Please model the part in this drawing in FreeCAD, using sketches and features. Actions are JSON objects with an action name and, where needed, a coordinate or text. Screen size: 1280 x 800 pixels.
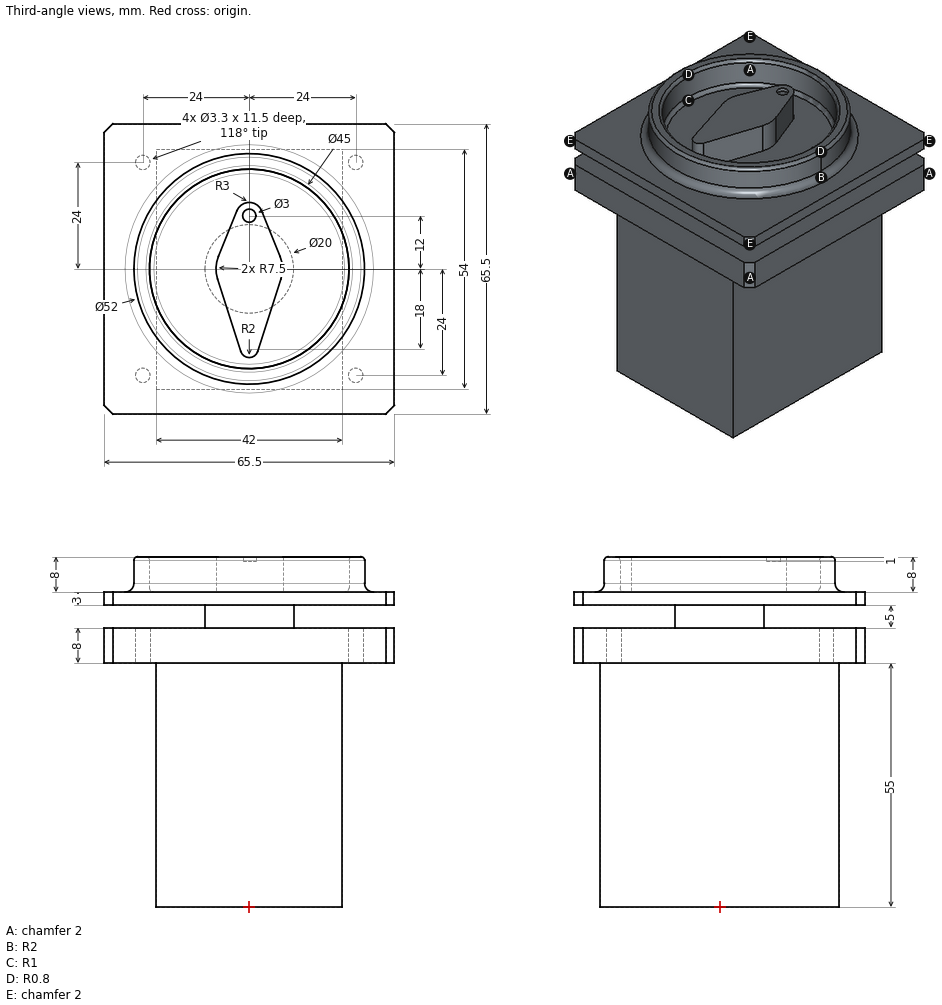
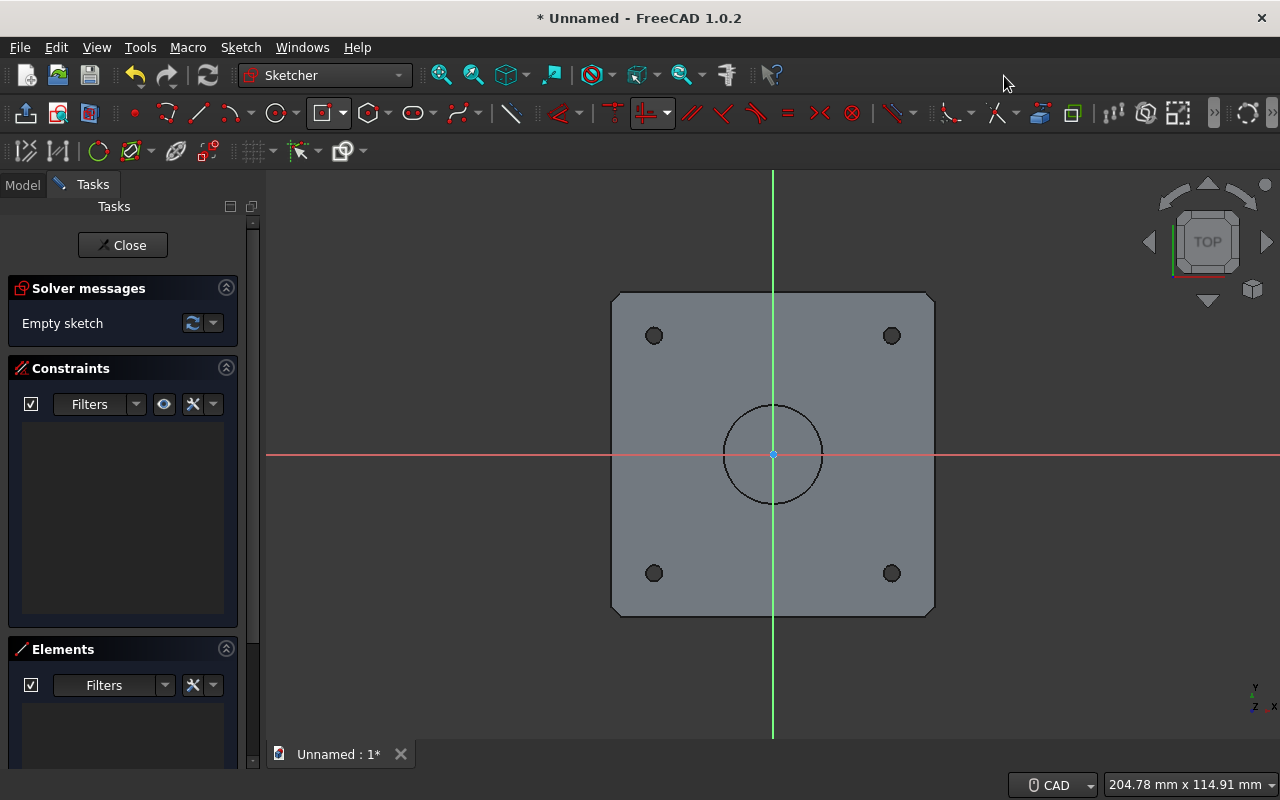
{"action": "left_click", "coordinate": [322, 114]}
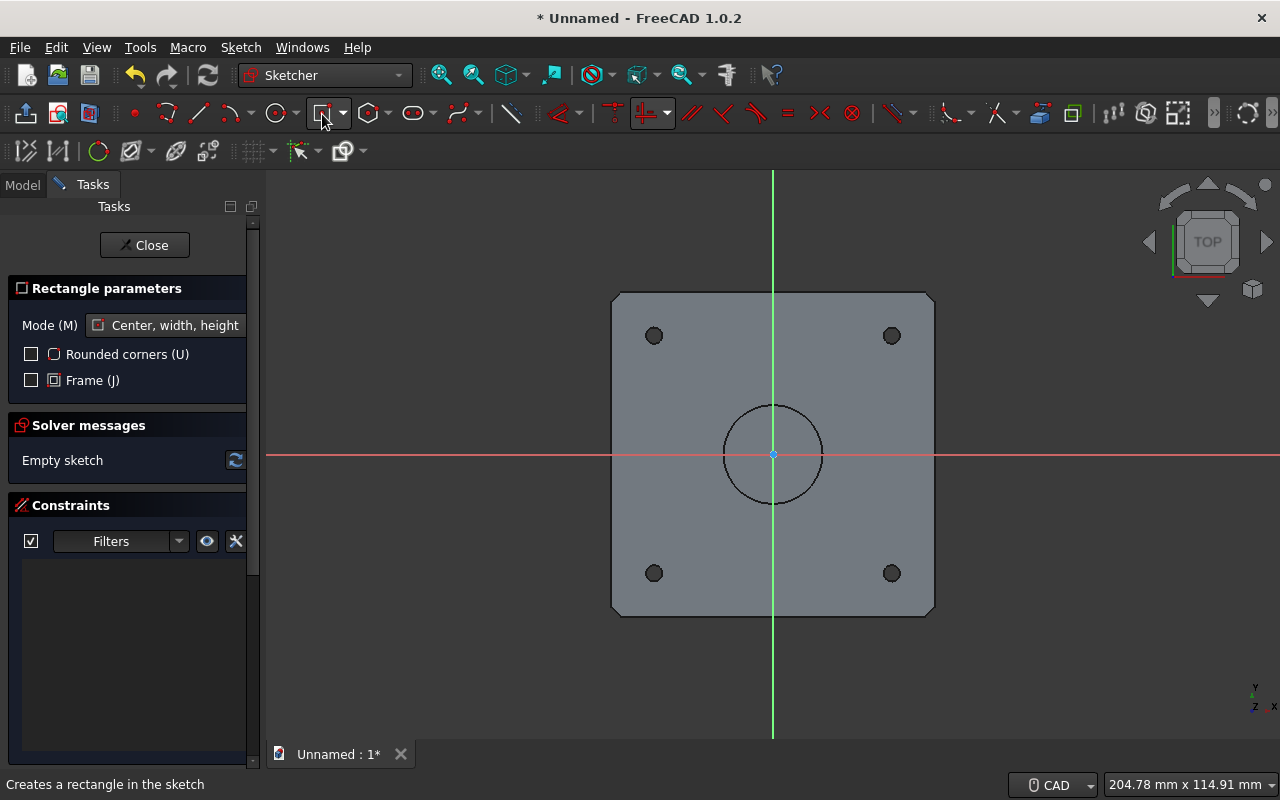
{"action": "left_click", "coordinate": [773, 455]}
{"action": "mouse_move", "coordinate": [935, 292]}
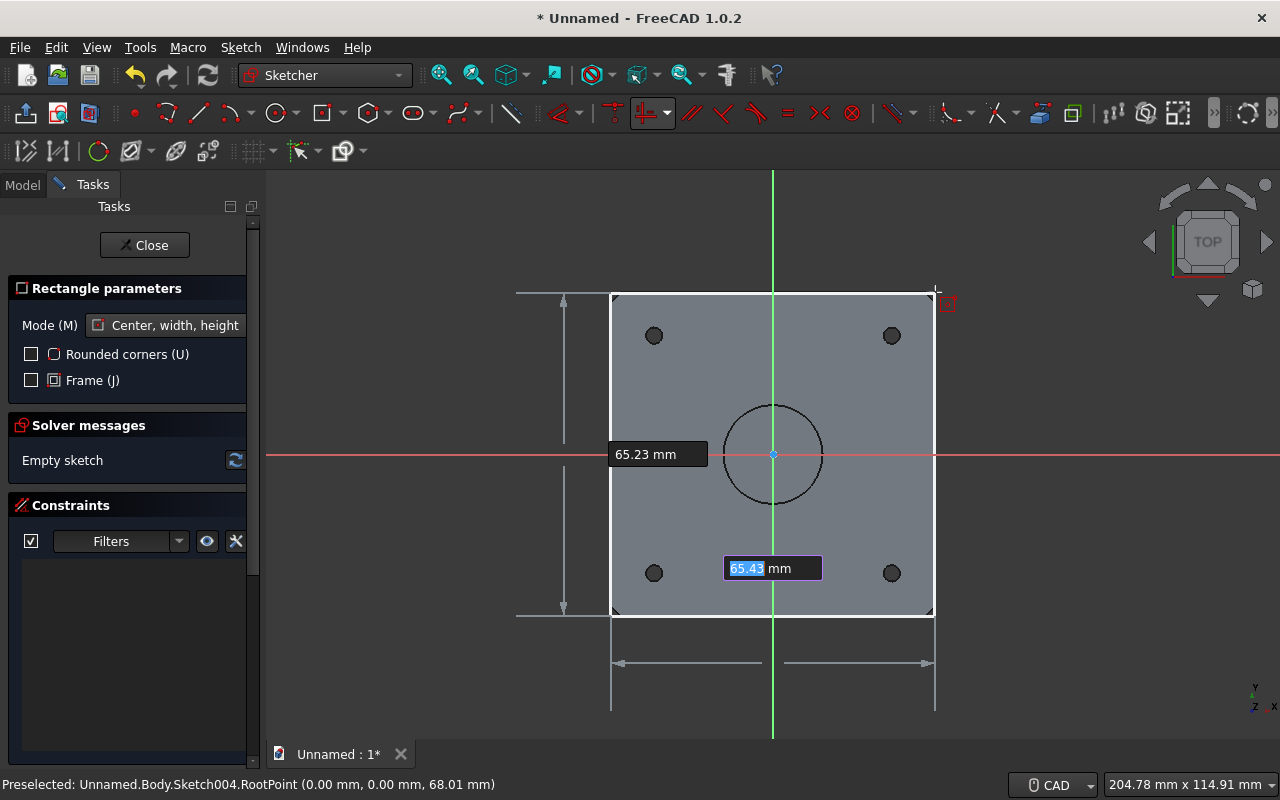
{"action": "type", "text": "65.5"}
{"action": "key", "text": "Tab"}
{"action": "type", "text": "65.5"}
{"action": "key", "text": "Return"}
{"action": "key", "text": "Escape"}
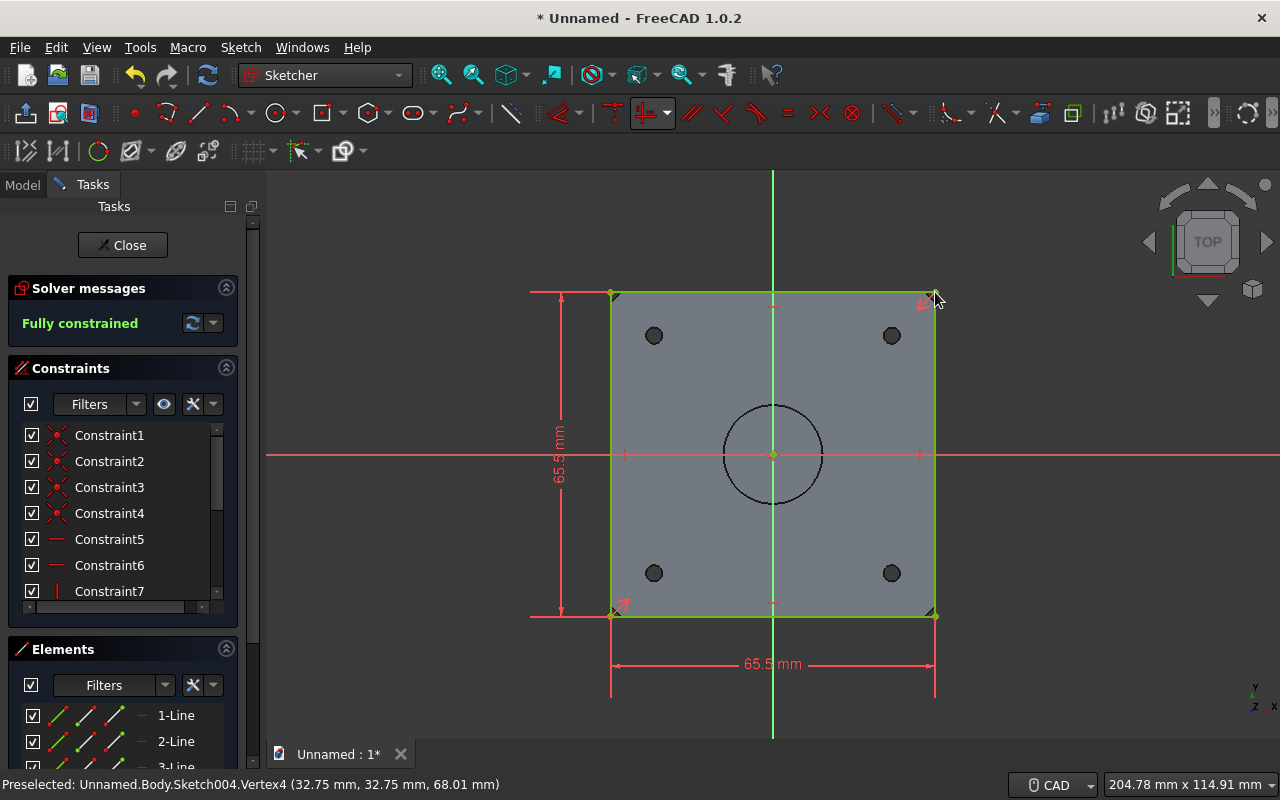
{"action": "left_click", "coordinate": [123, 245]}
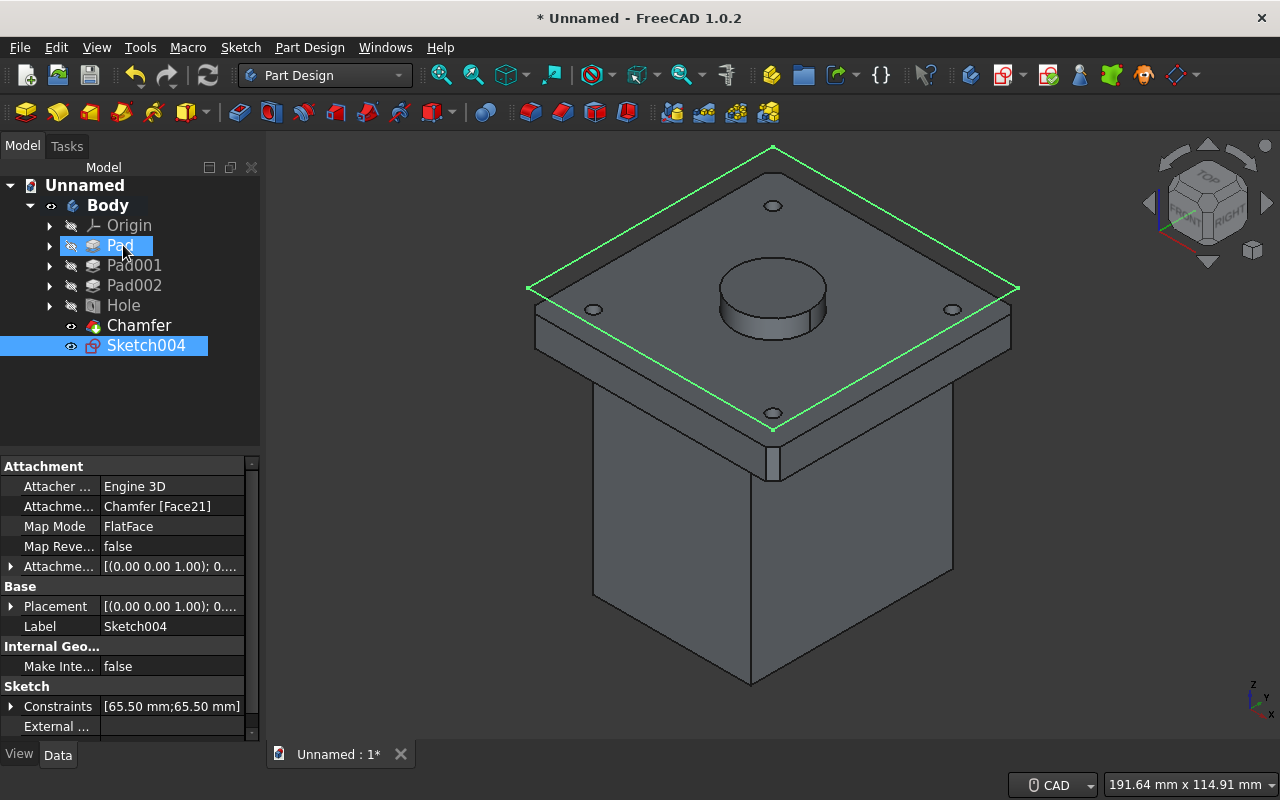
{"action": "left_click", "coordinate": [26, 112]}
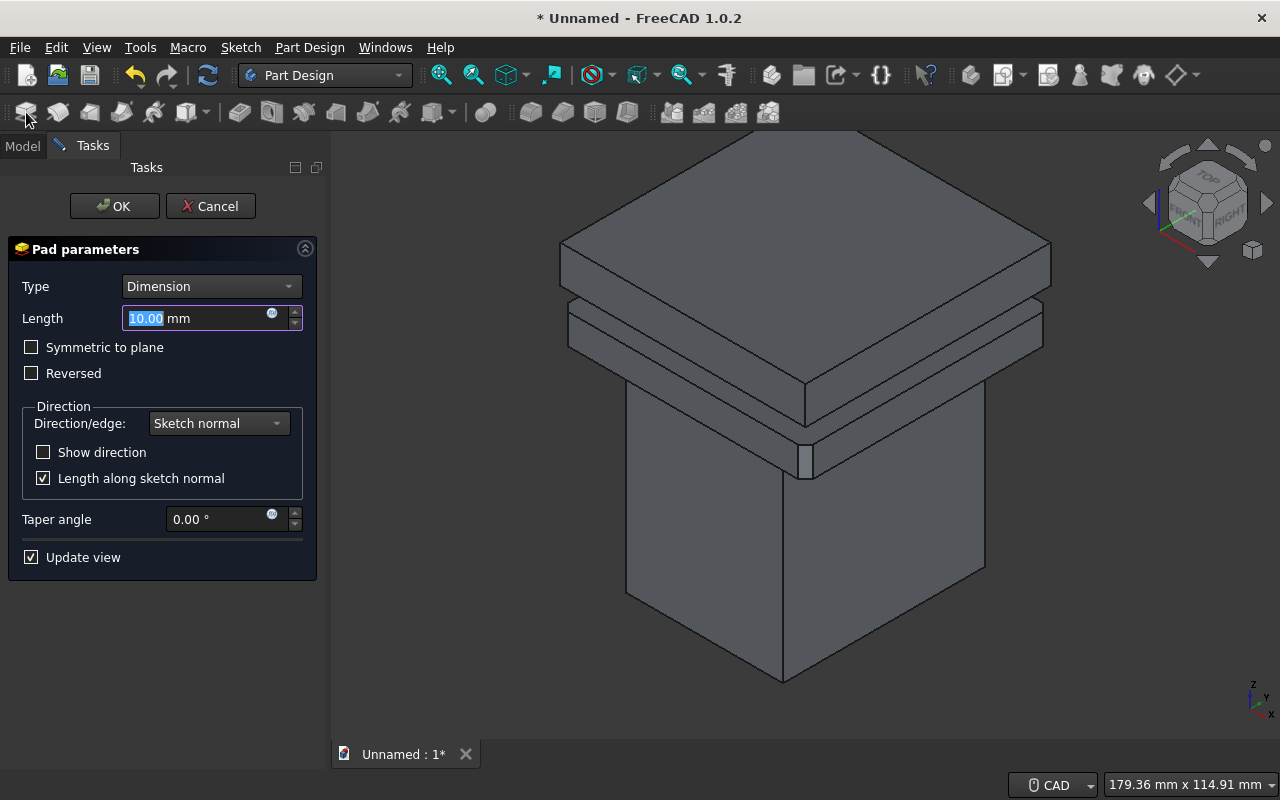
{"action": "type", "text": "3"}
{"action": "key", "text": "Tab"}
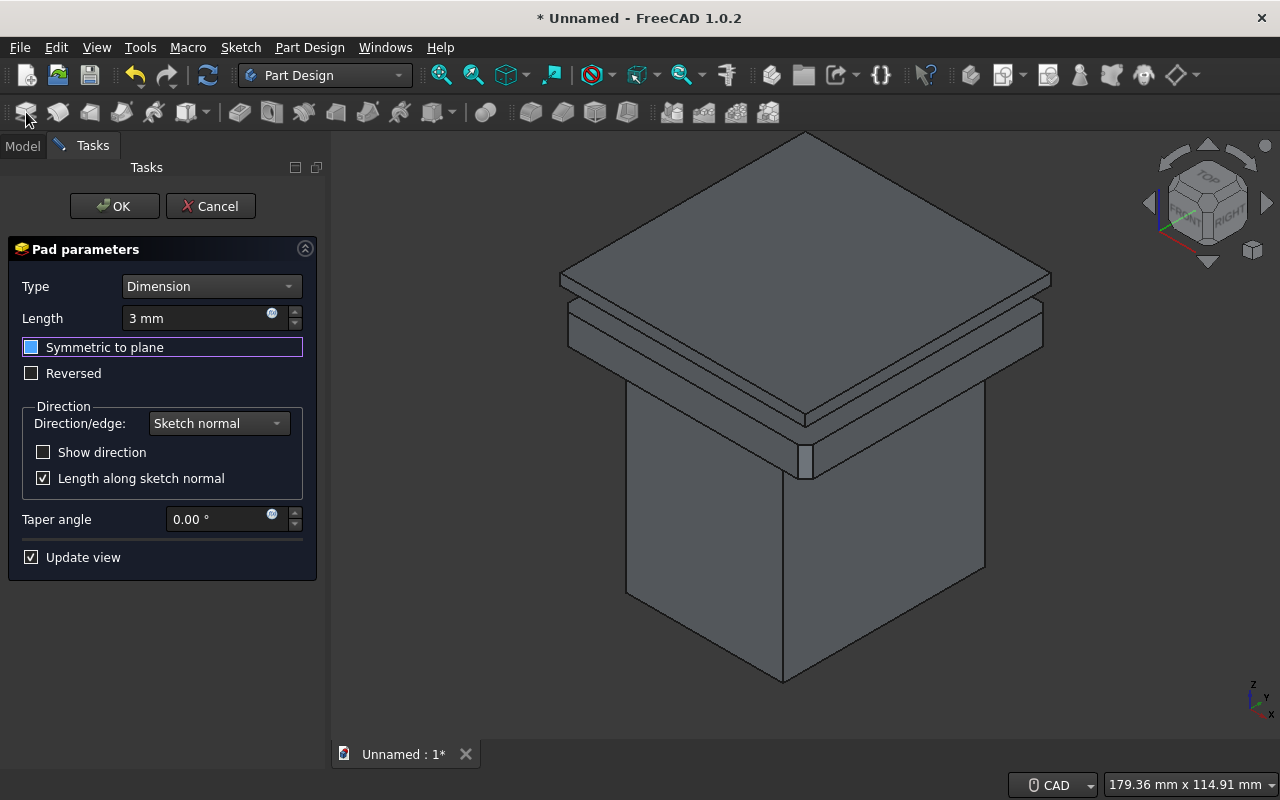
{"action": "left_click", "coordinate": [115, 206]}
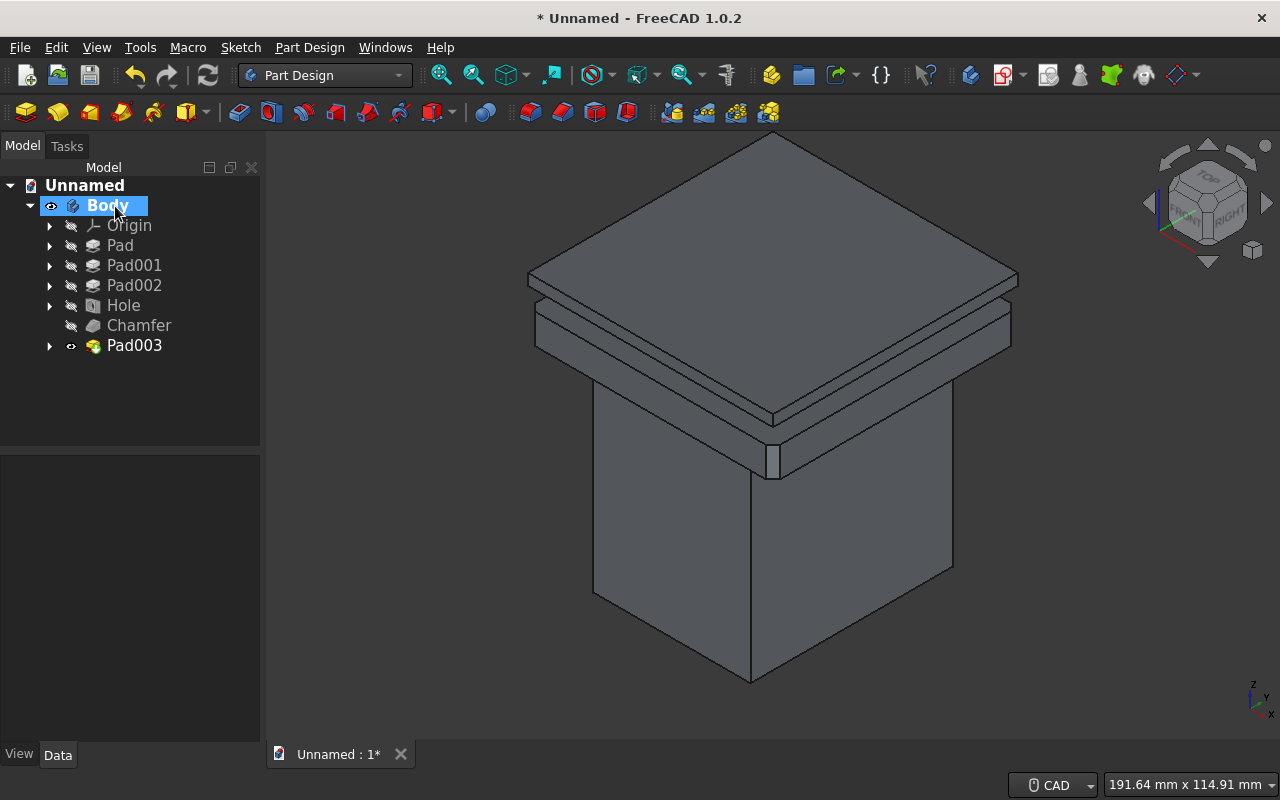
{"action": "left_click", "coordinate": [442, 76]}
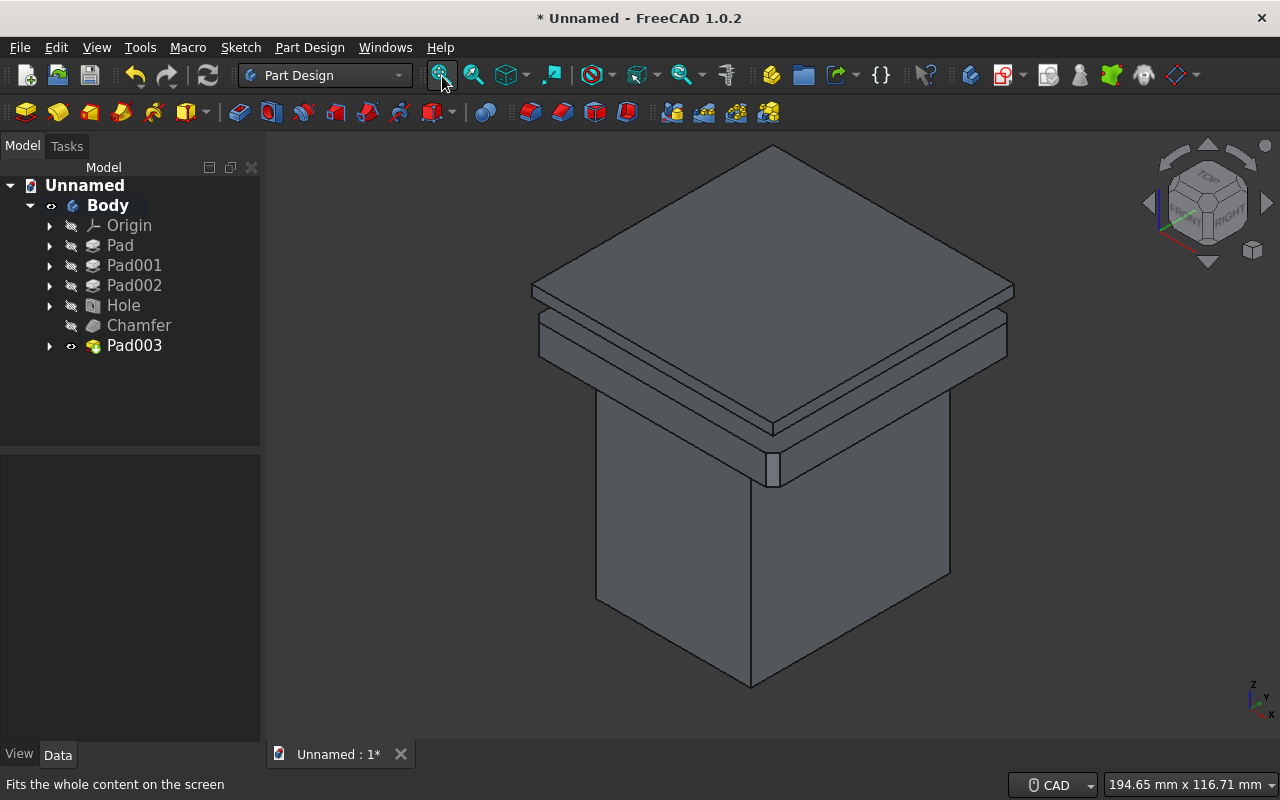
{"action": "left_click", "coordinate": [773, 283]}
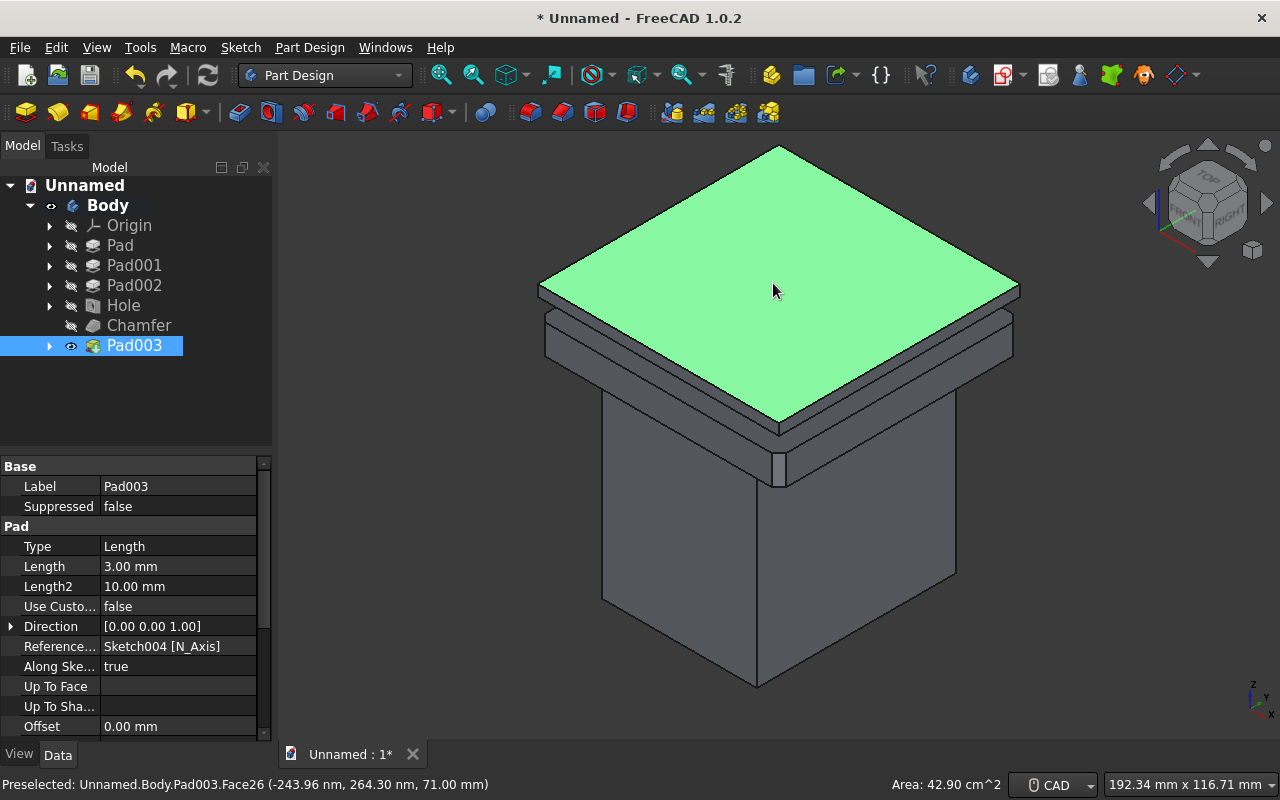
{"action": "left_click", "coordinate": [1004, 76]}